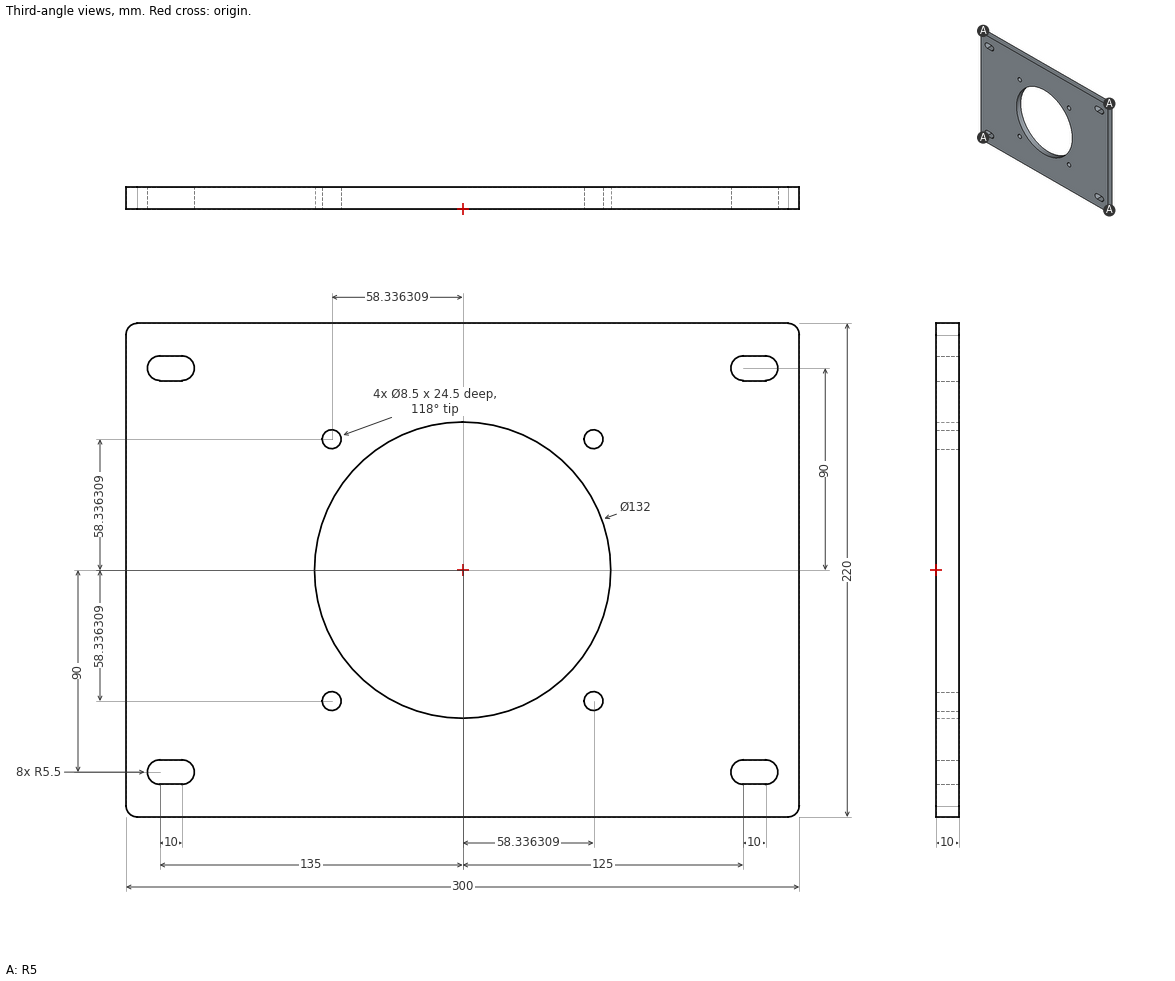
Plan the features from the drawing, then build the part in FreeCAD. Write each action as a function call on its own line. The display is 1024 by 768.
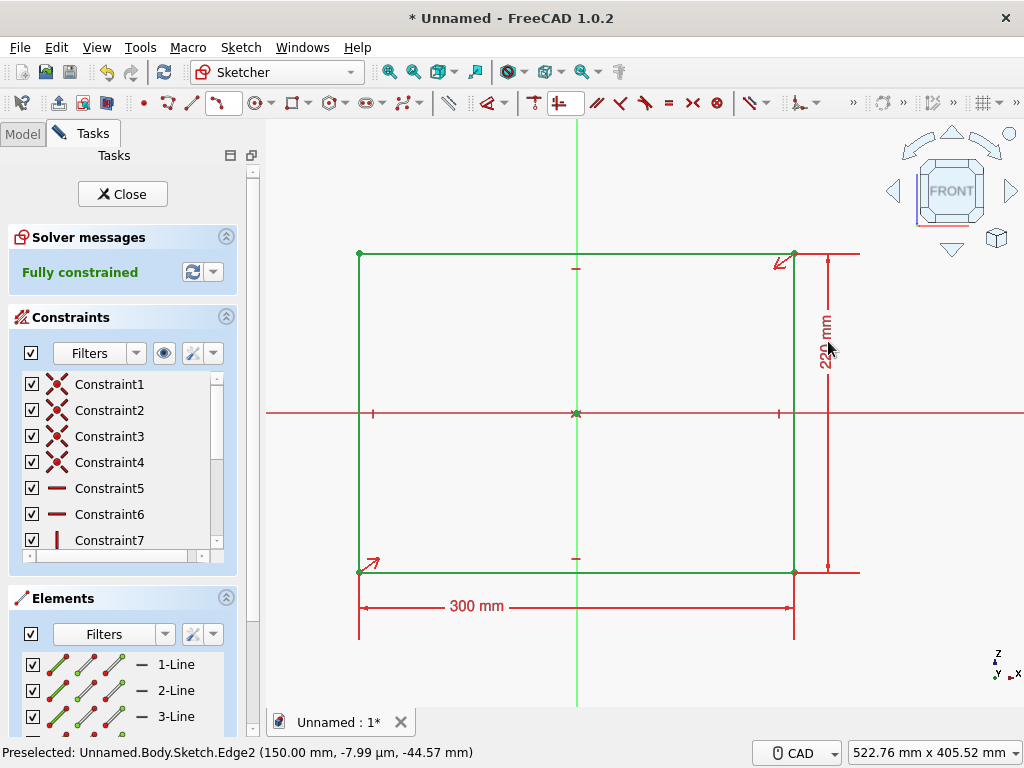
click(123, 194)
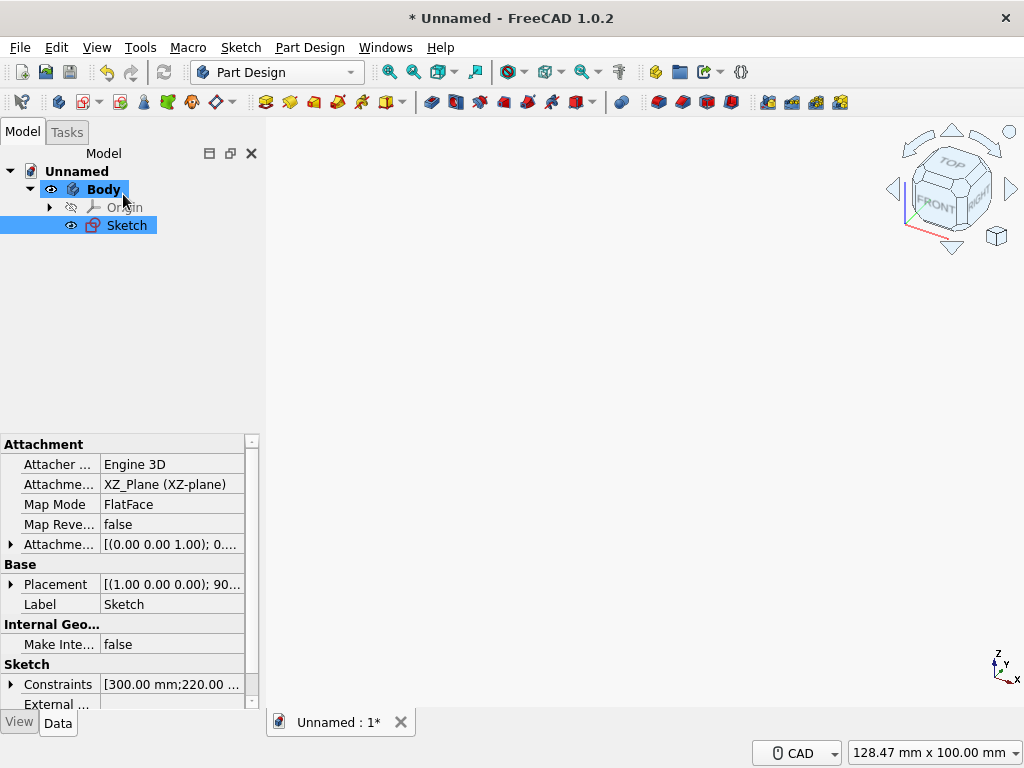
click(266, 102)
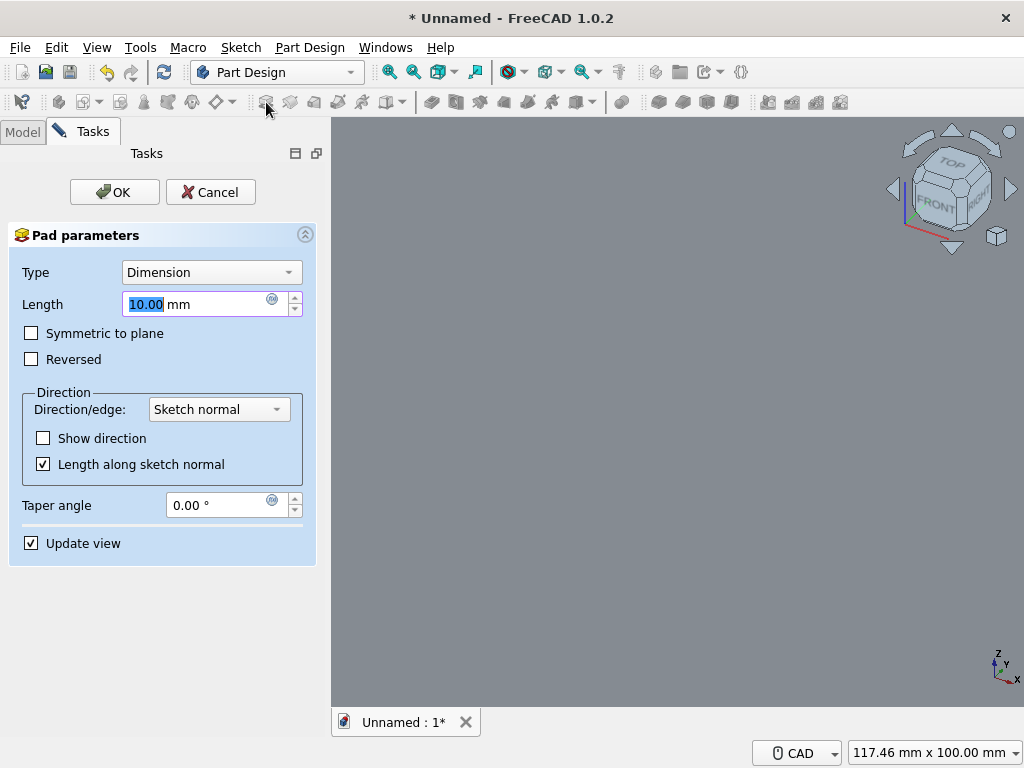
text(10)
key(Tab)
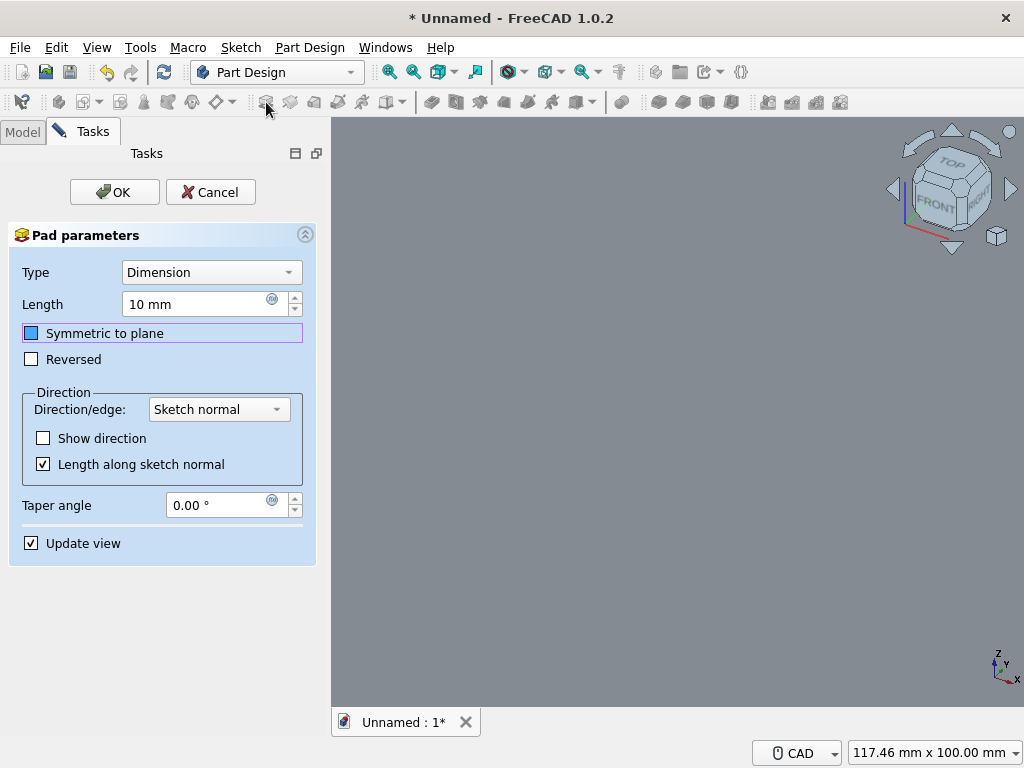
click(30, 359)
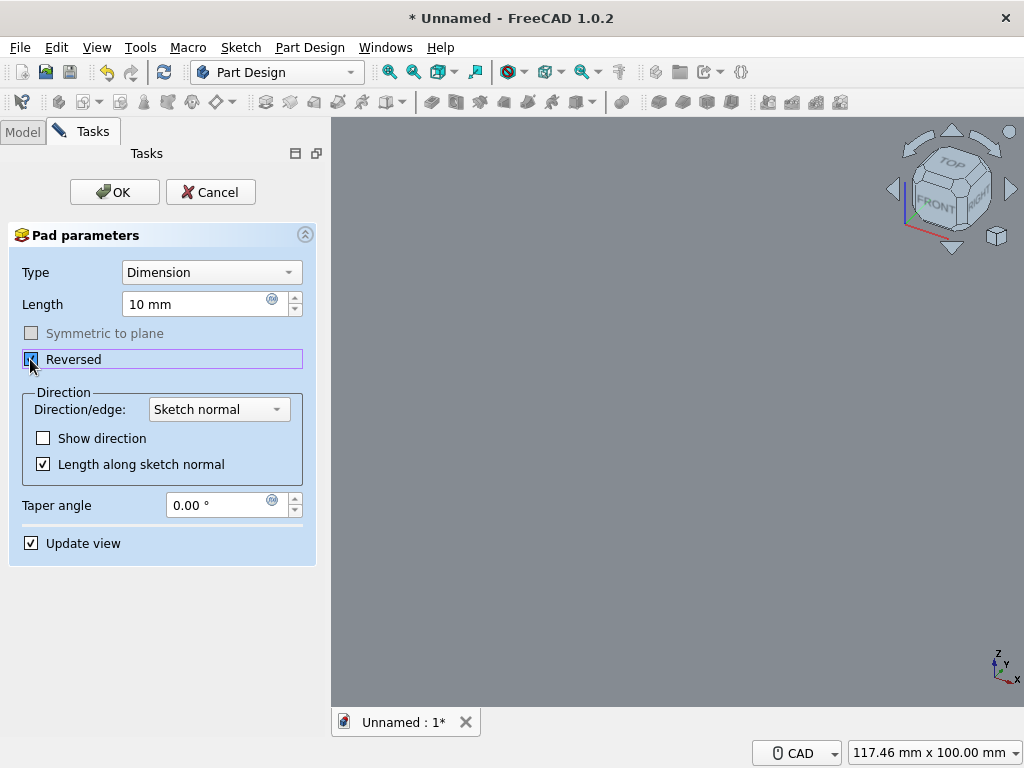
click(115, 192)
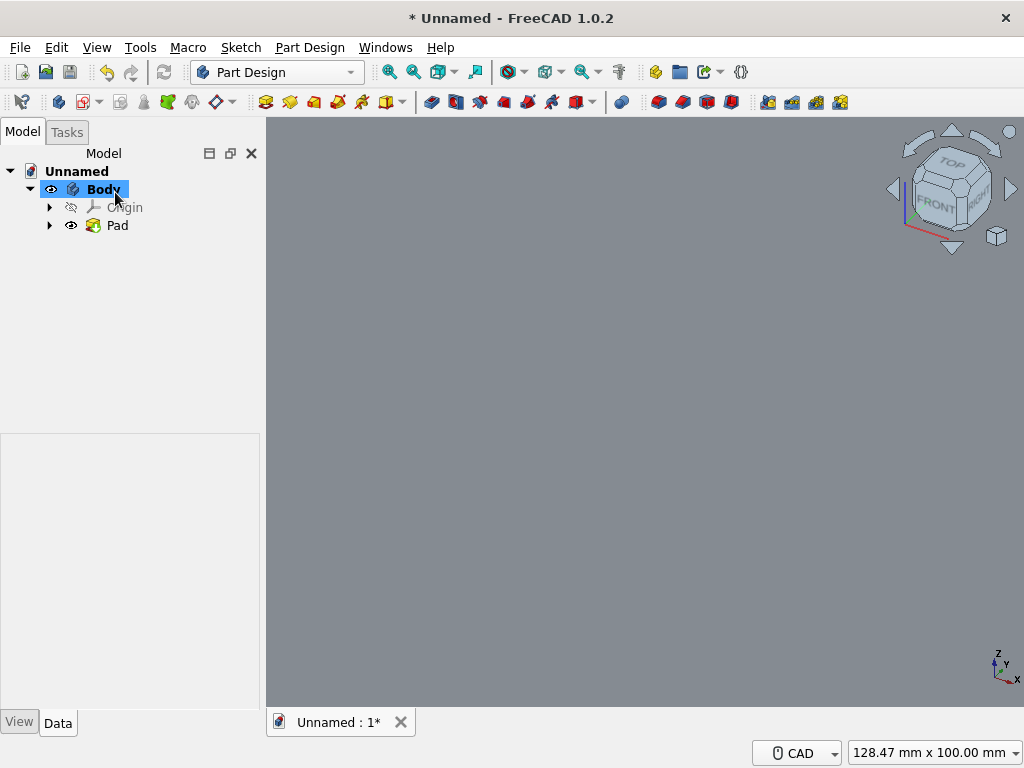
key(v)
key(f)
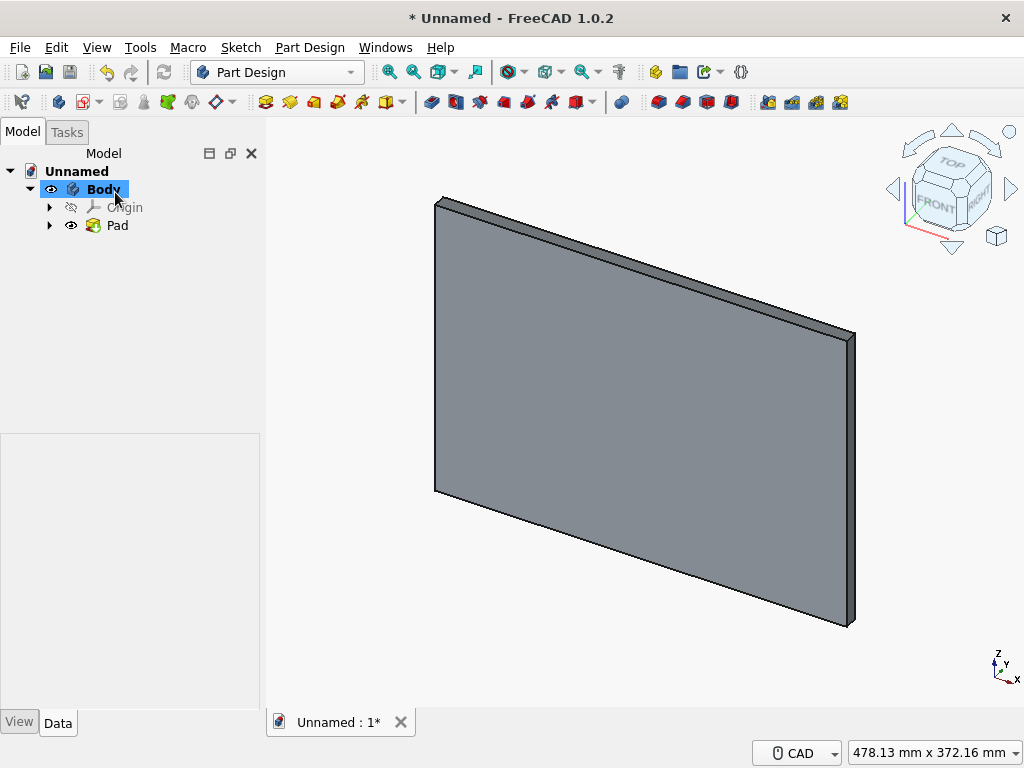
key(4)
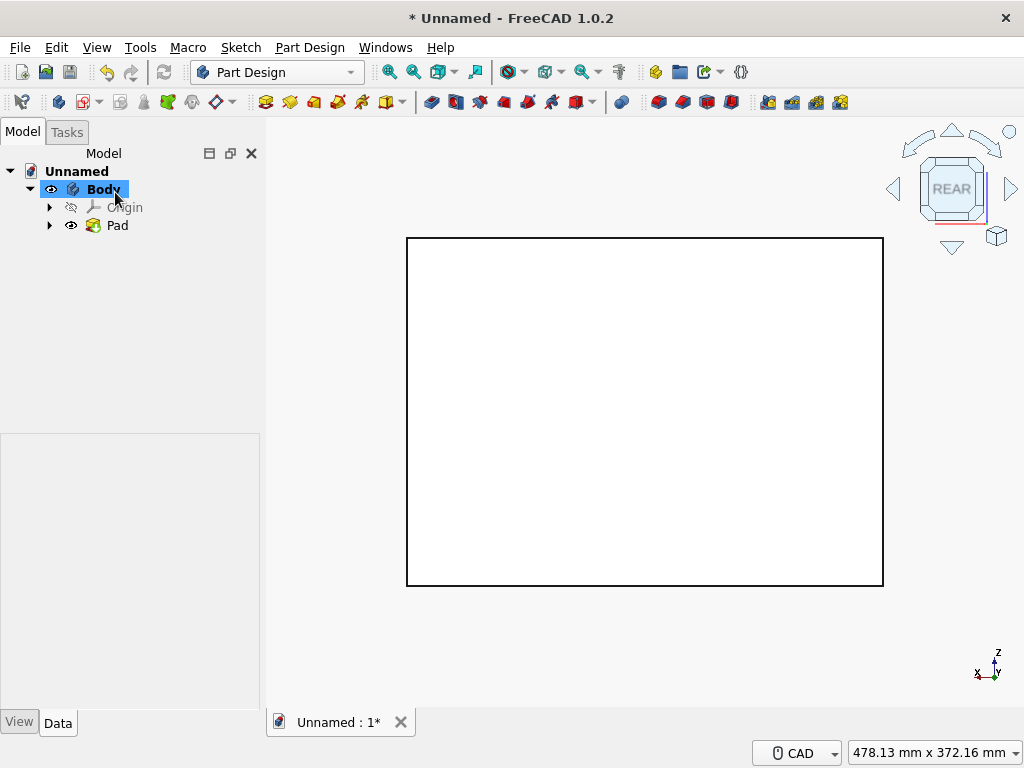
click(645, 411)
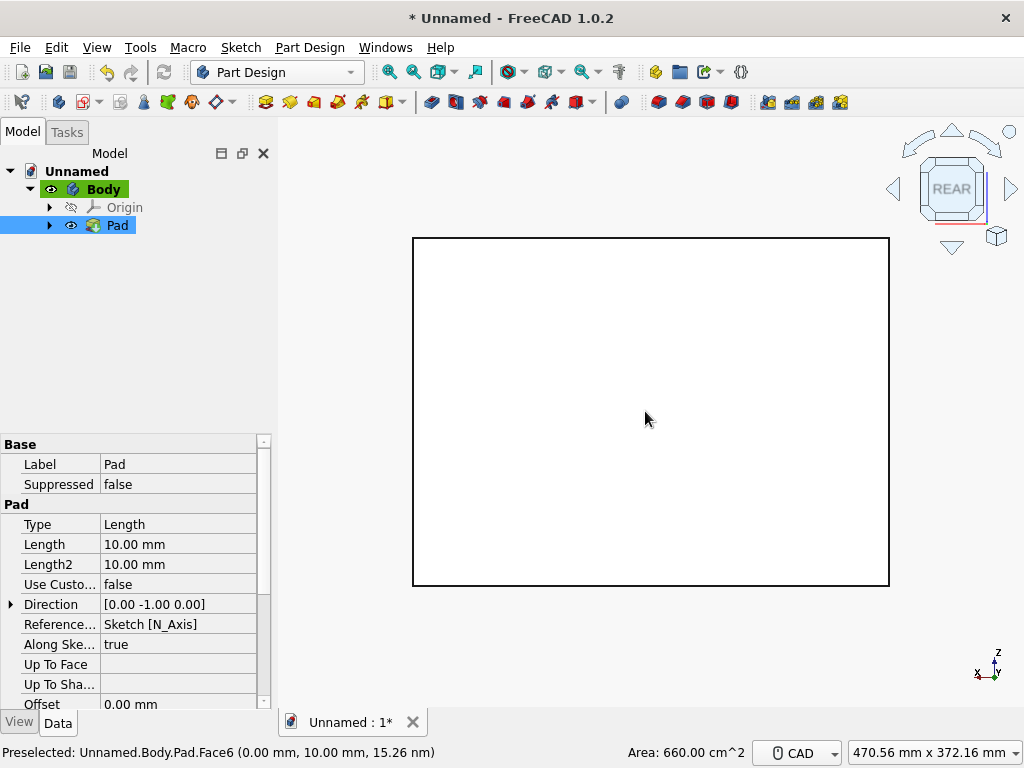
click(84, 102)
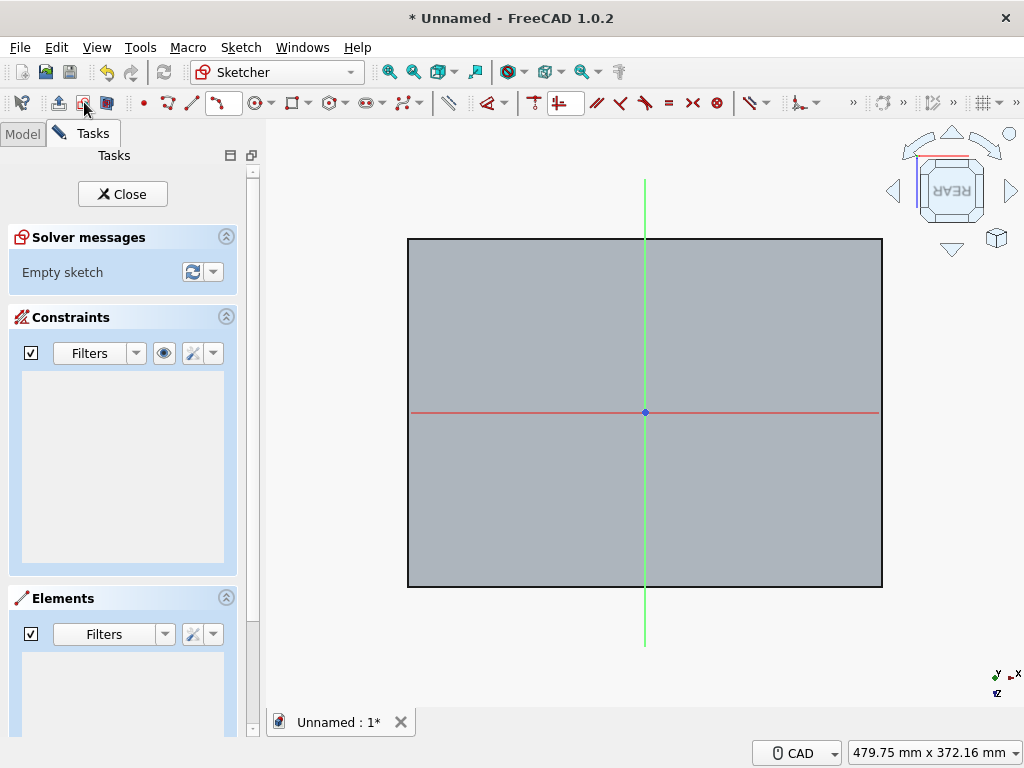
scroll(728, 413, up, 3)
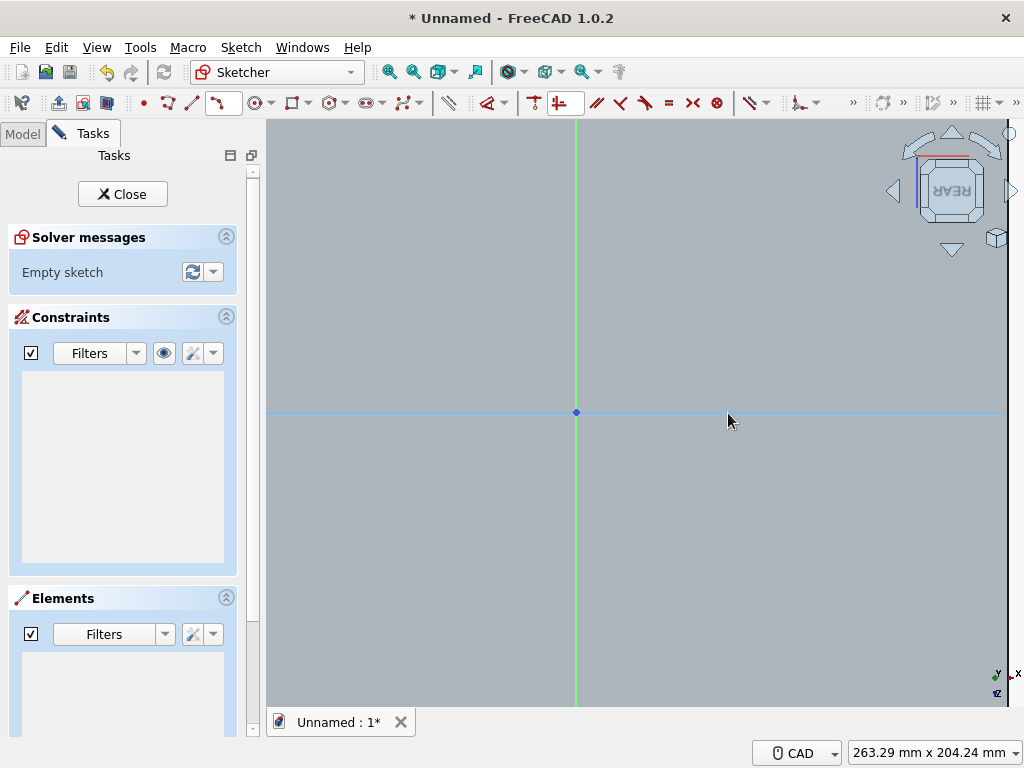
key(g)
key(c)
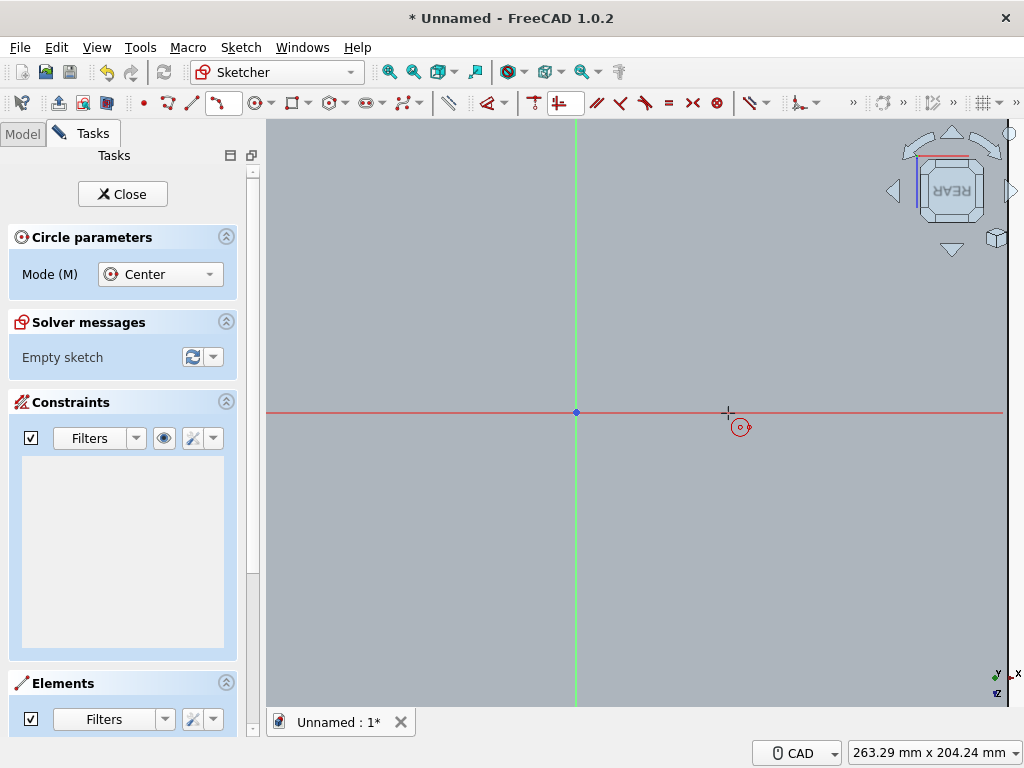
click(576, 413)
click(711, 278)
key(Escape)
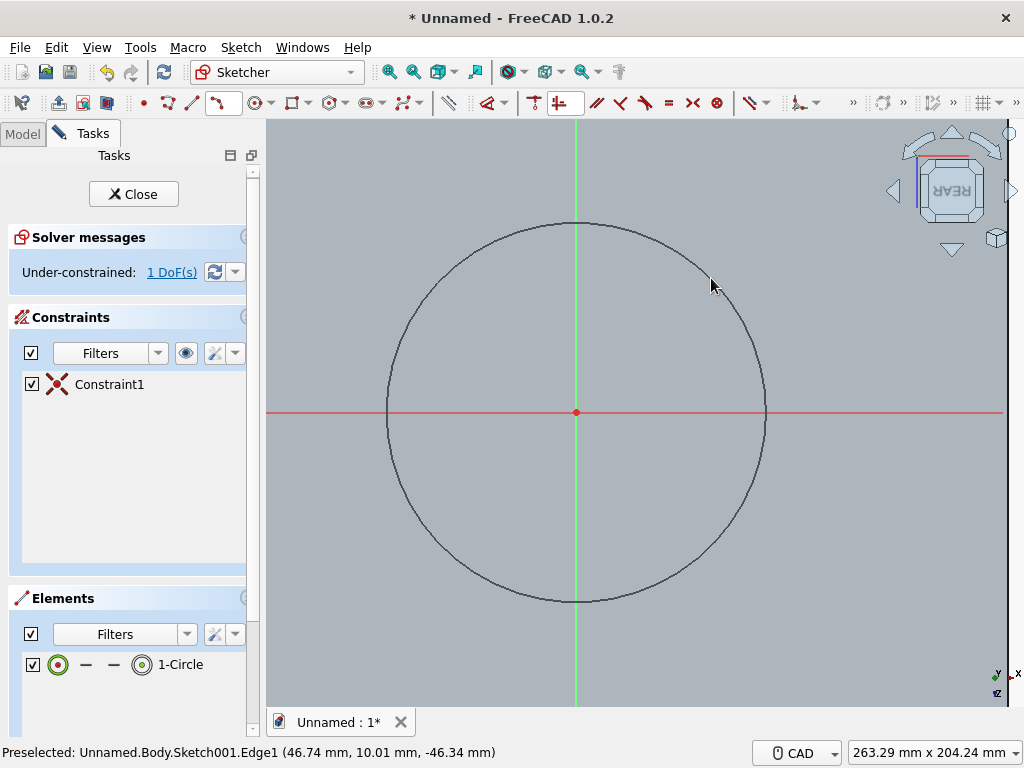
key(d)